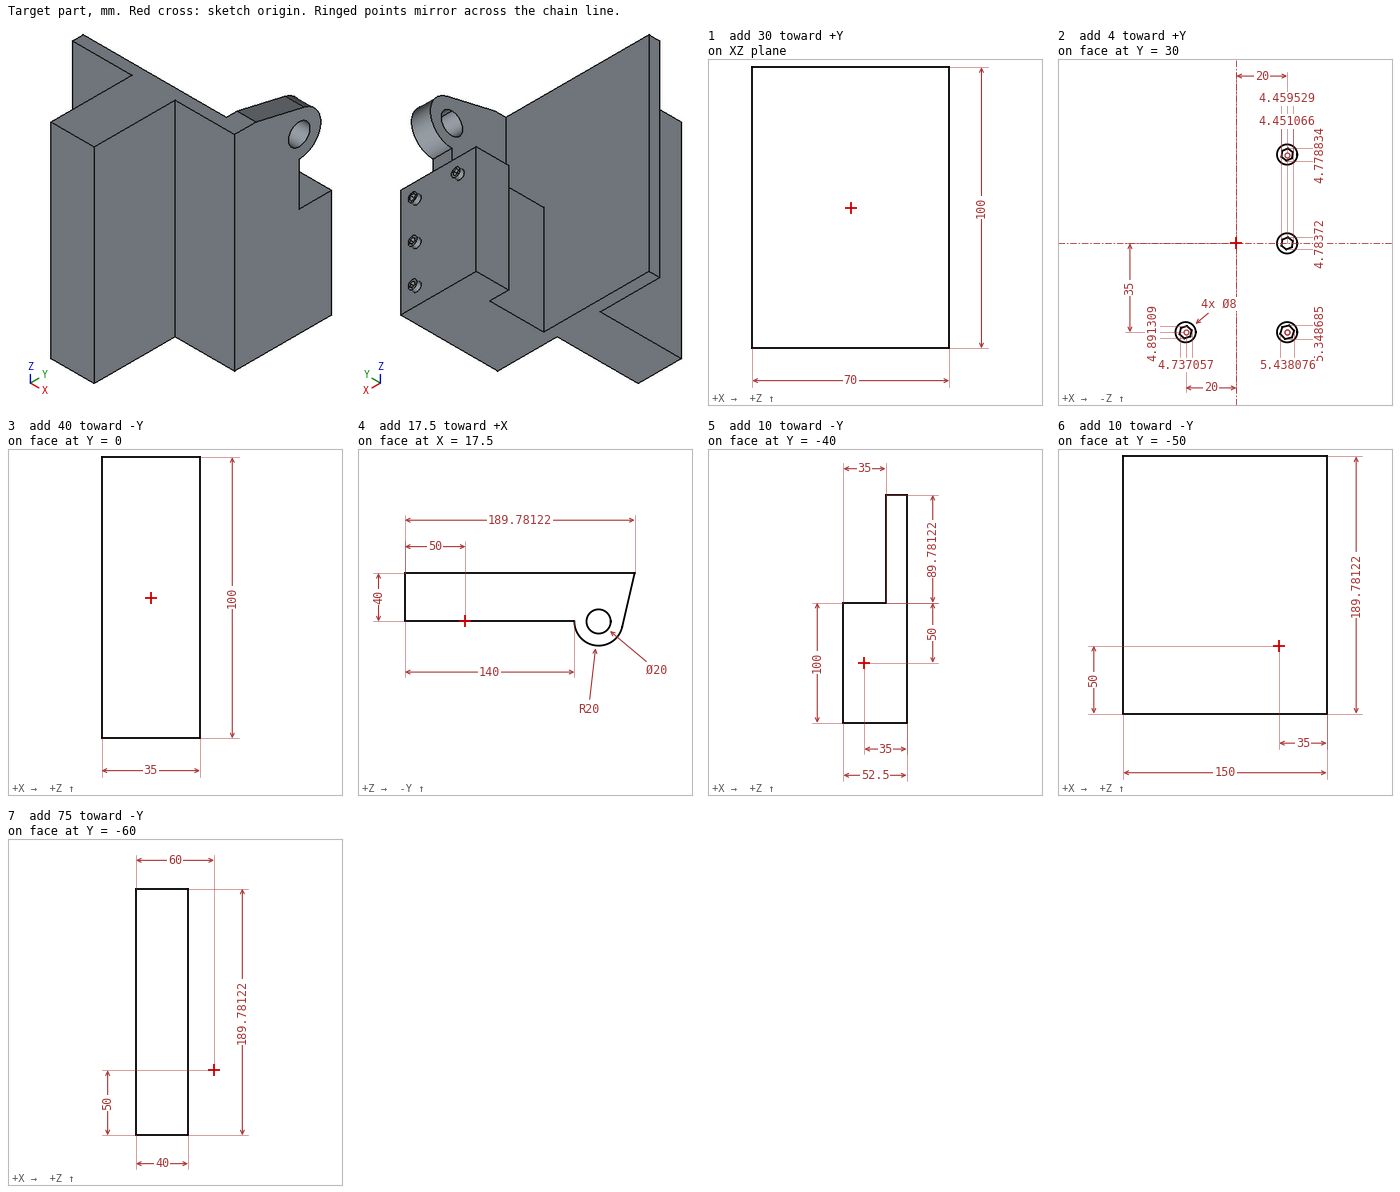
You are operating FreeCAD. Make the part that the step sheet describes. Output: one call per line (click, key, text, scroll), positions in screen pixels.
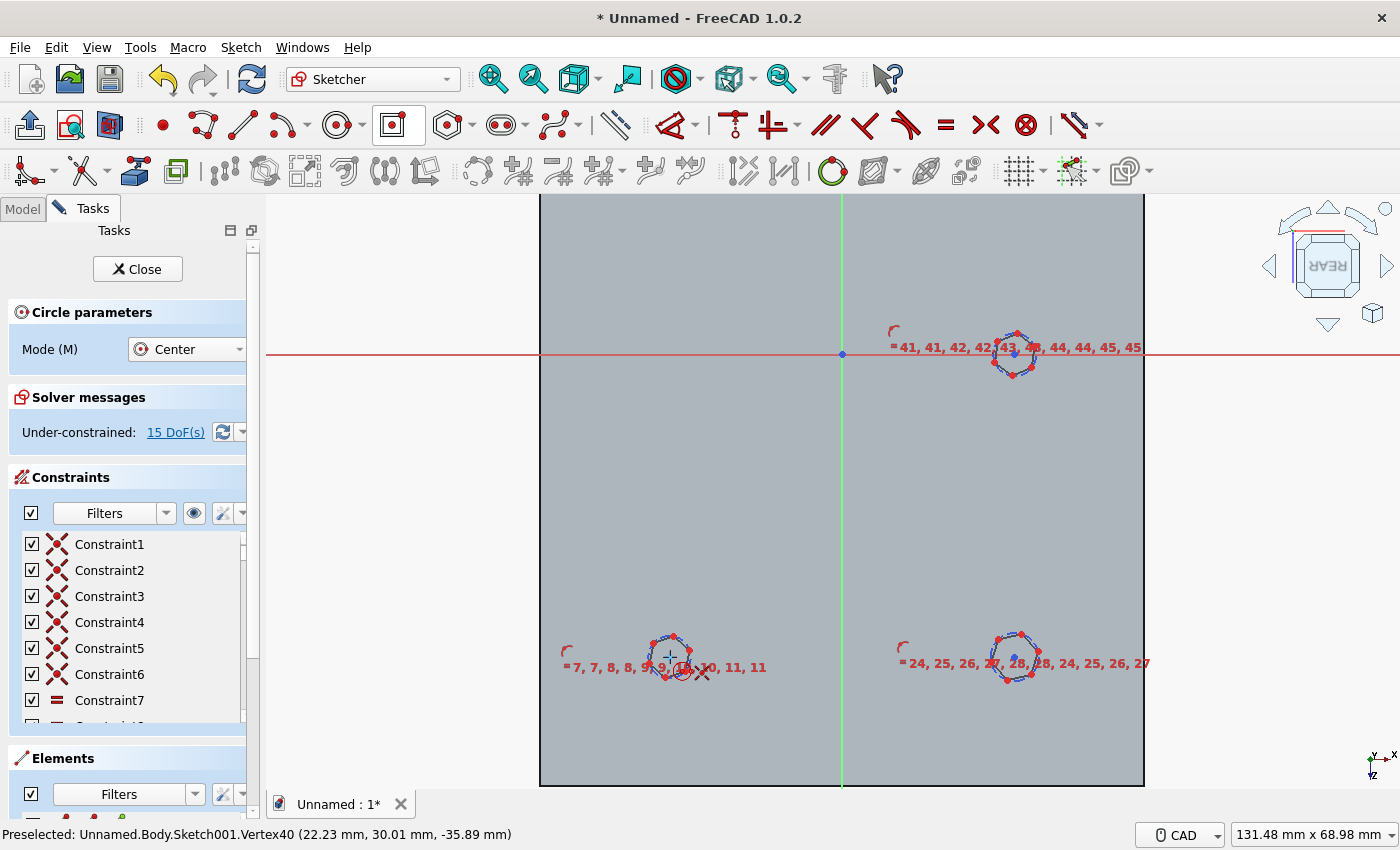
click(670, 657)
move(694, 632)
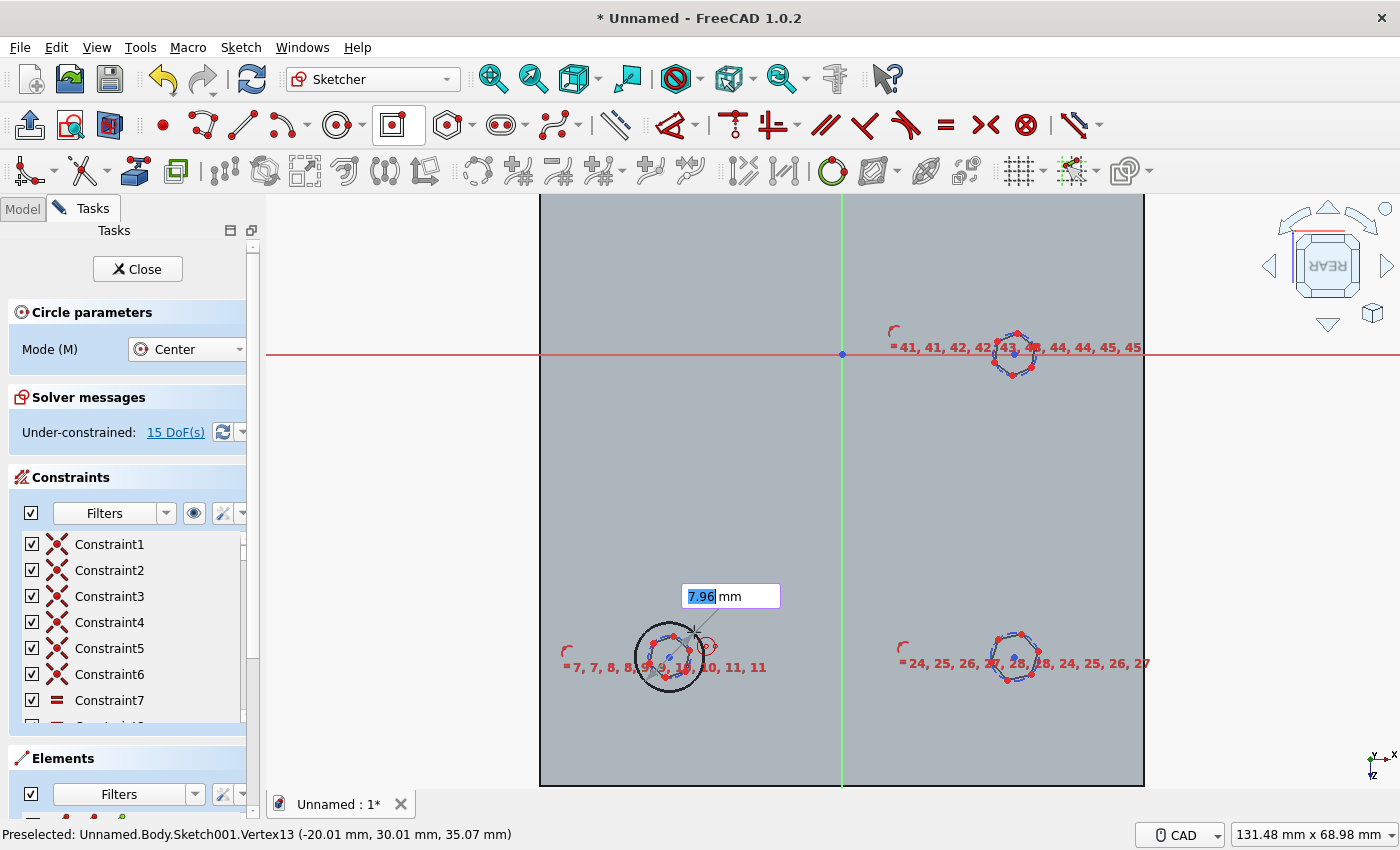
text(8)
key(Return)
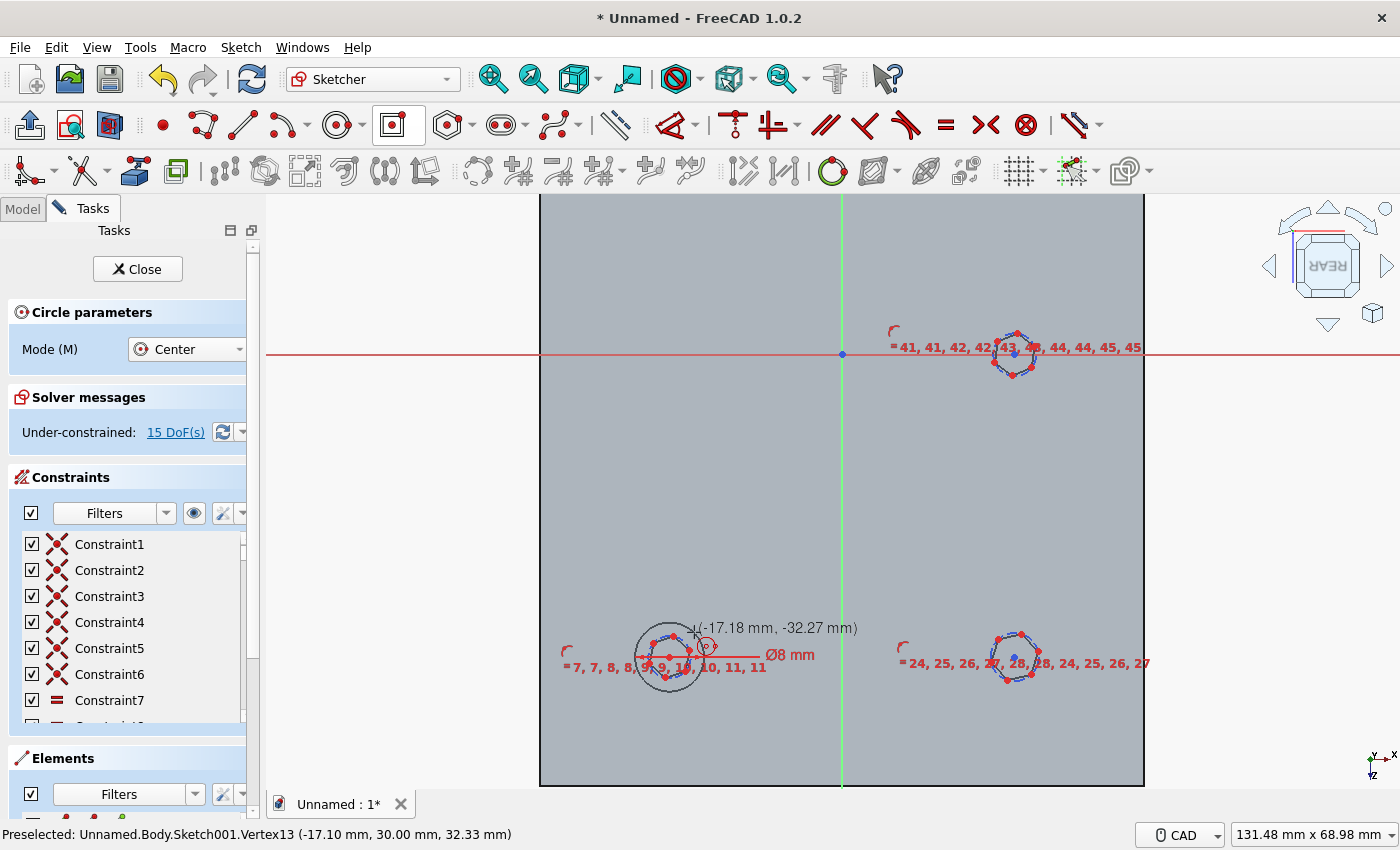
click(1015, 657)
move(1039, 632)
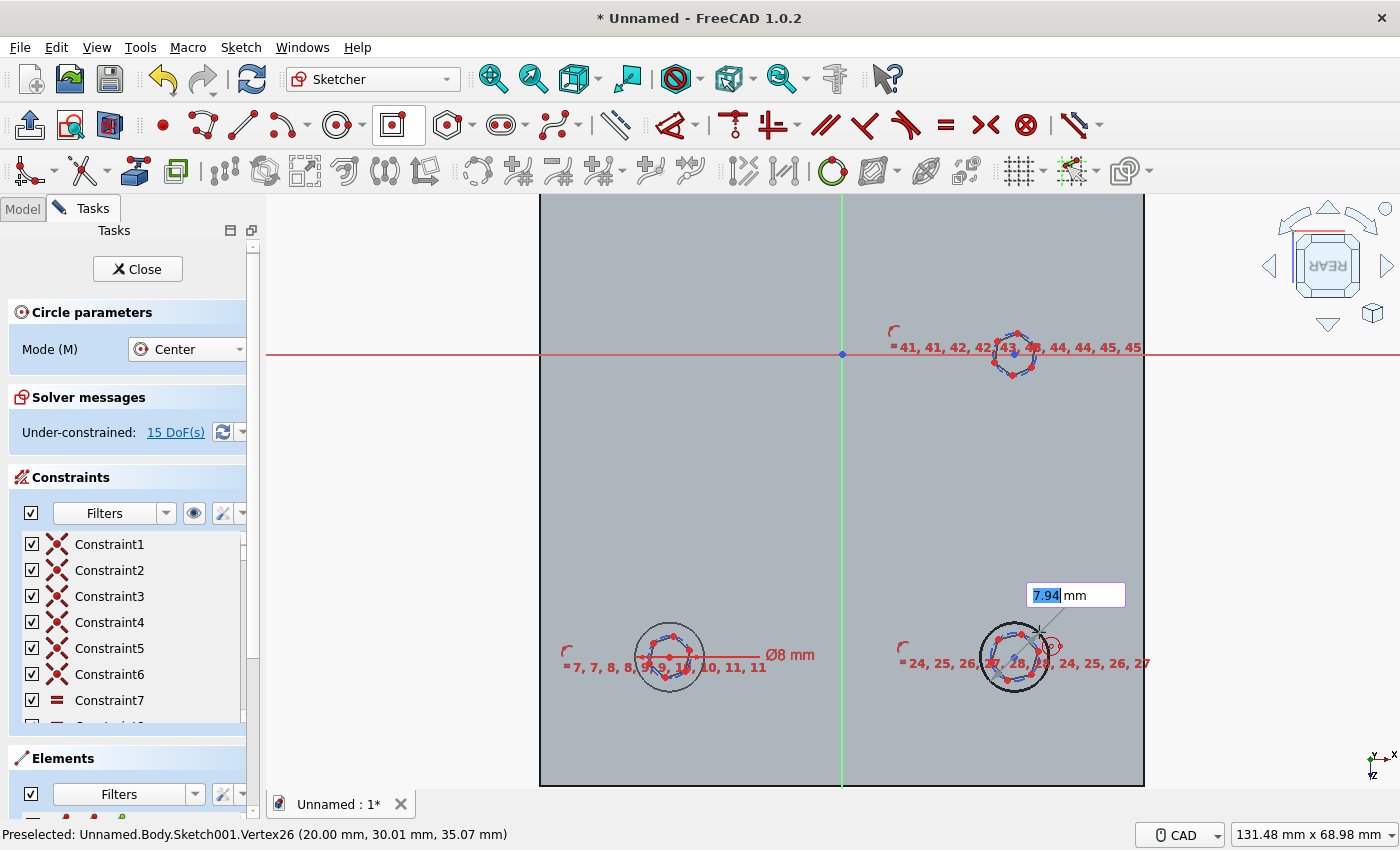
text(8)
key(Return)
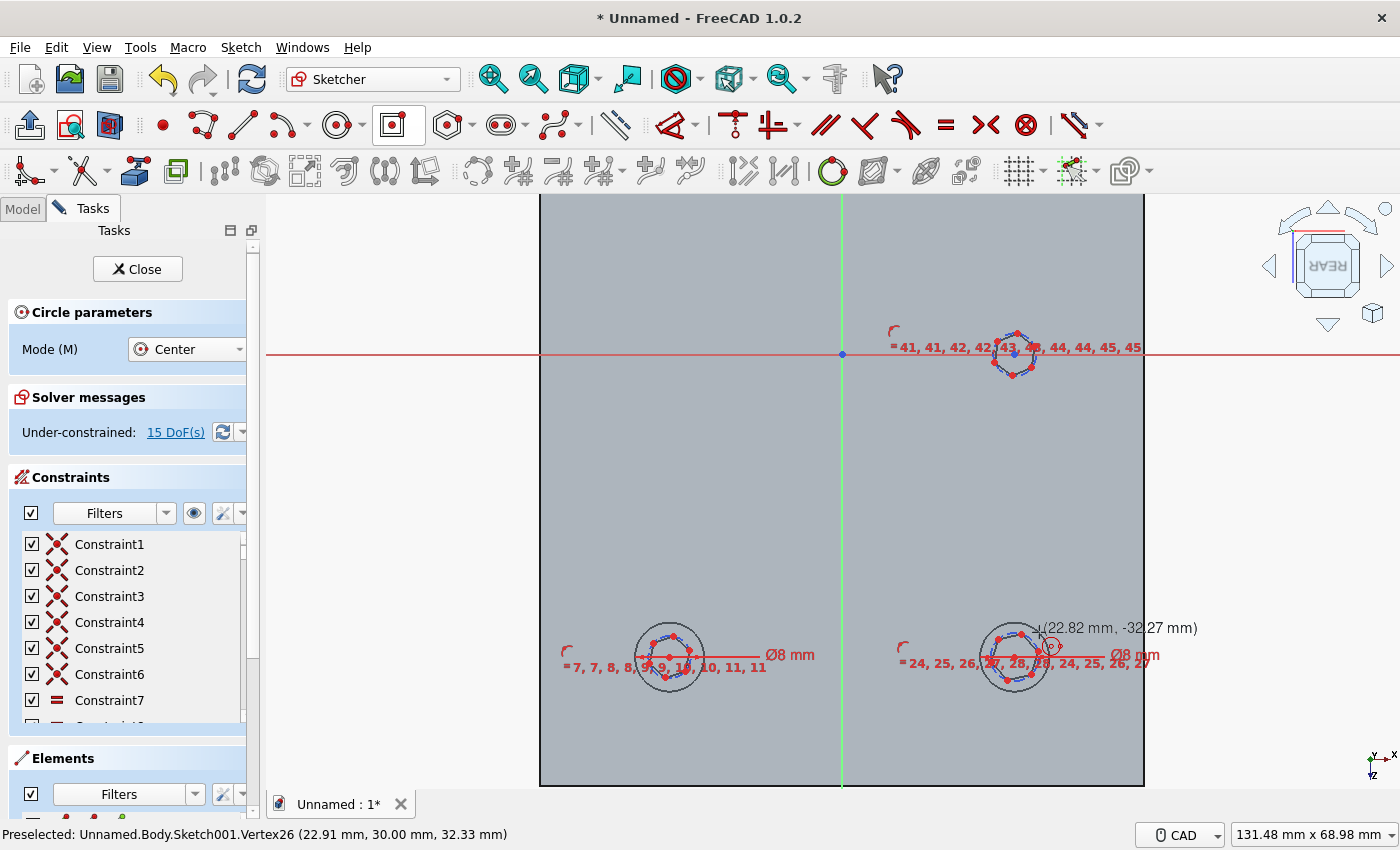
click(1015, 355)
move(1039, 330)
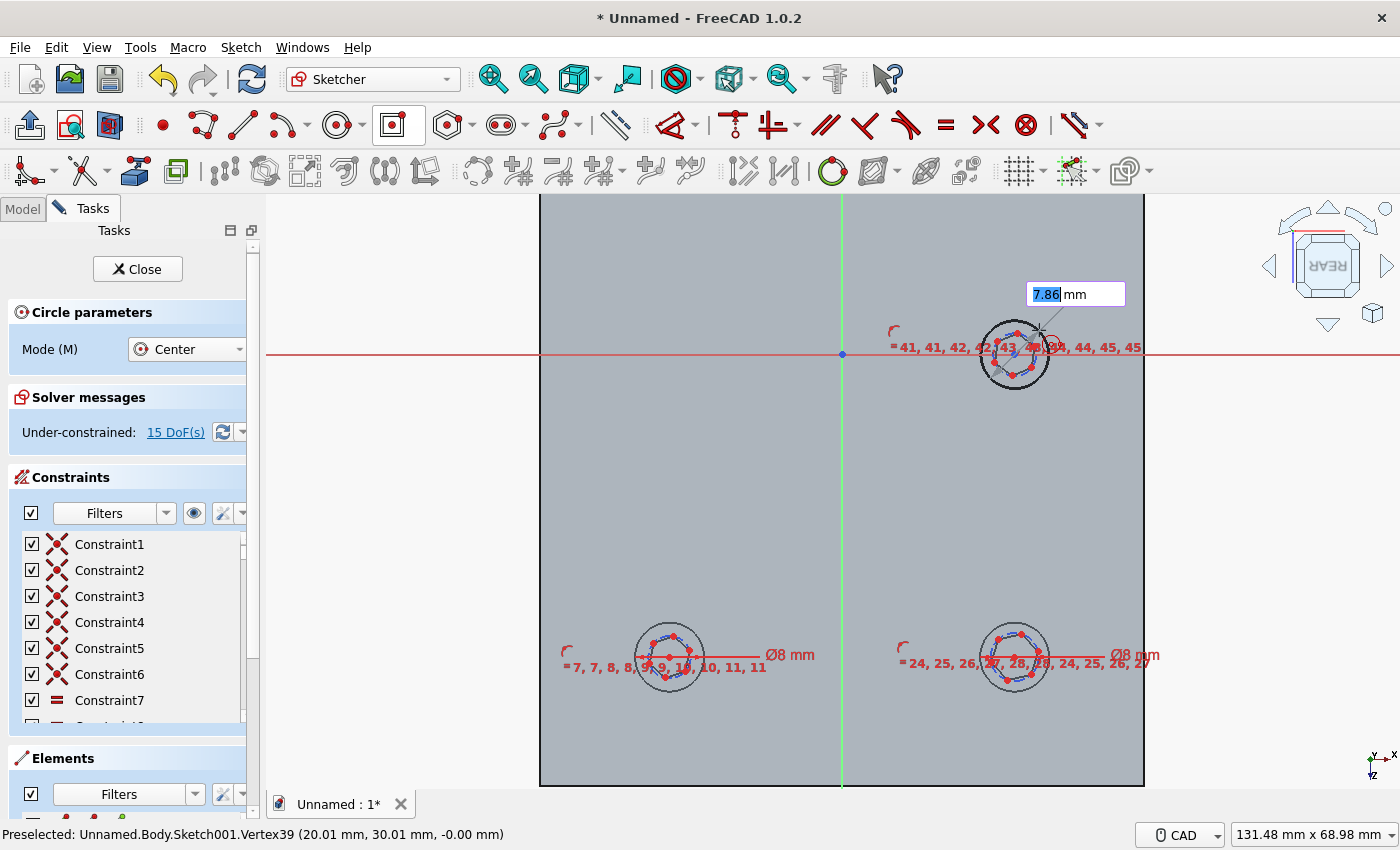
text(8)
key(Return)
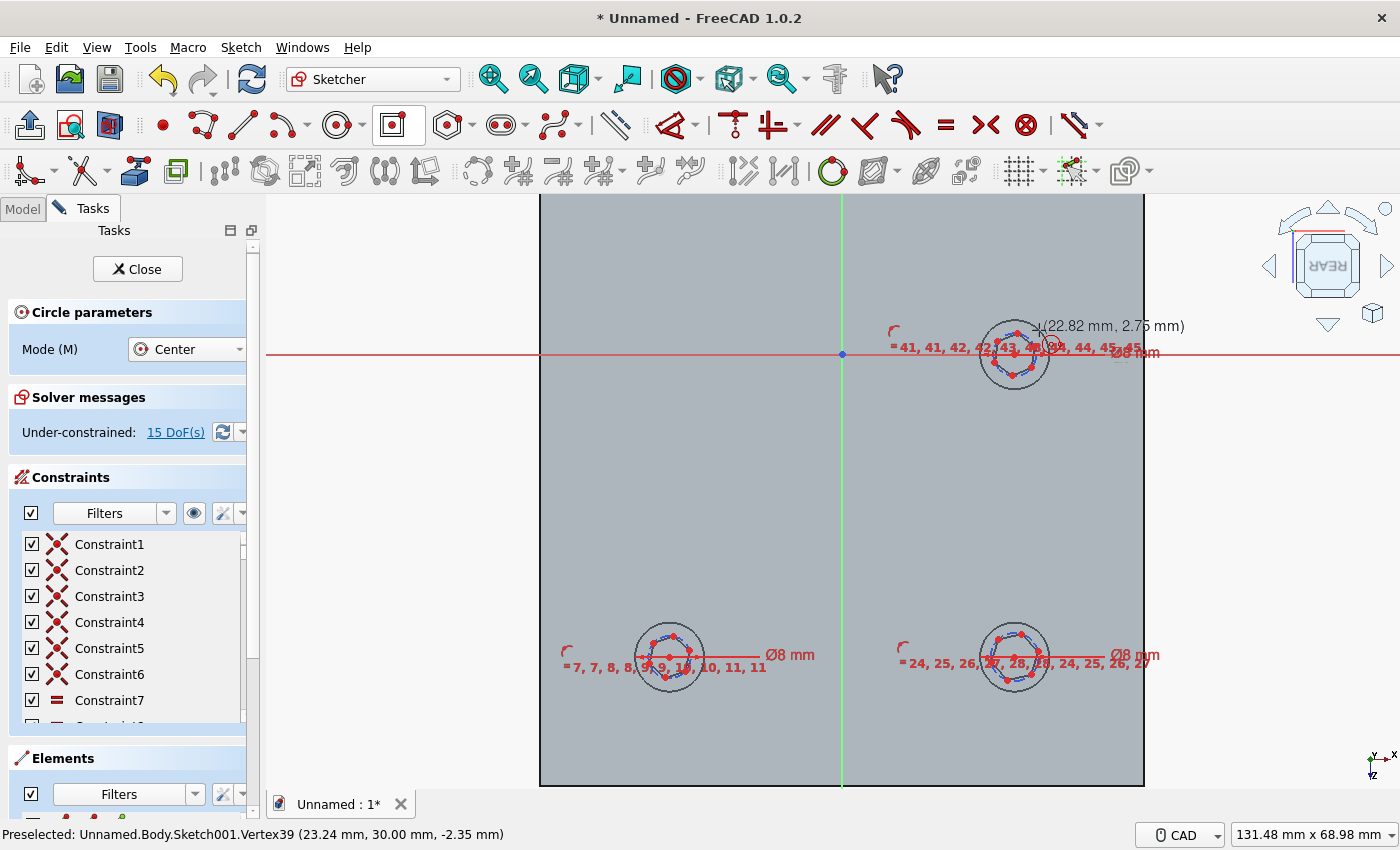
scroll(670, 658, down, 3)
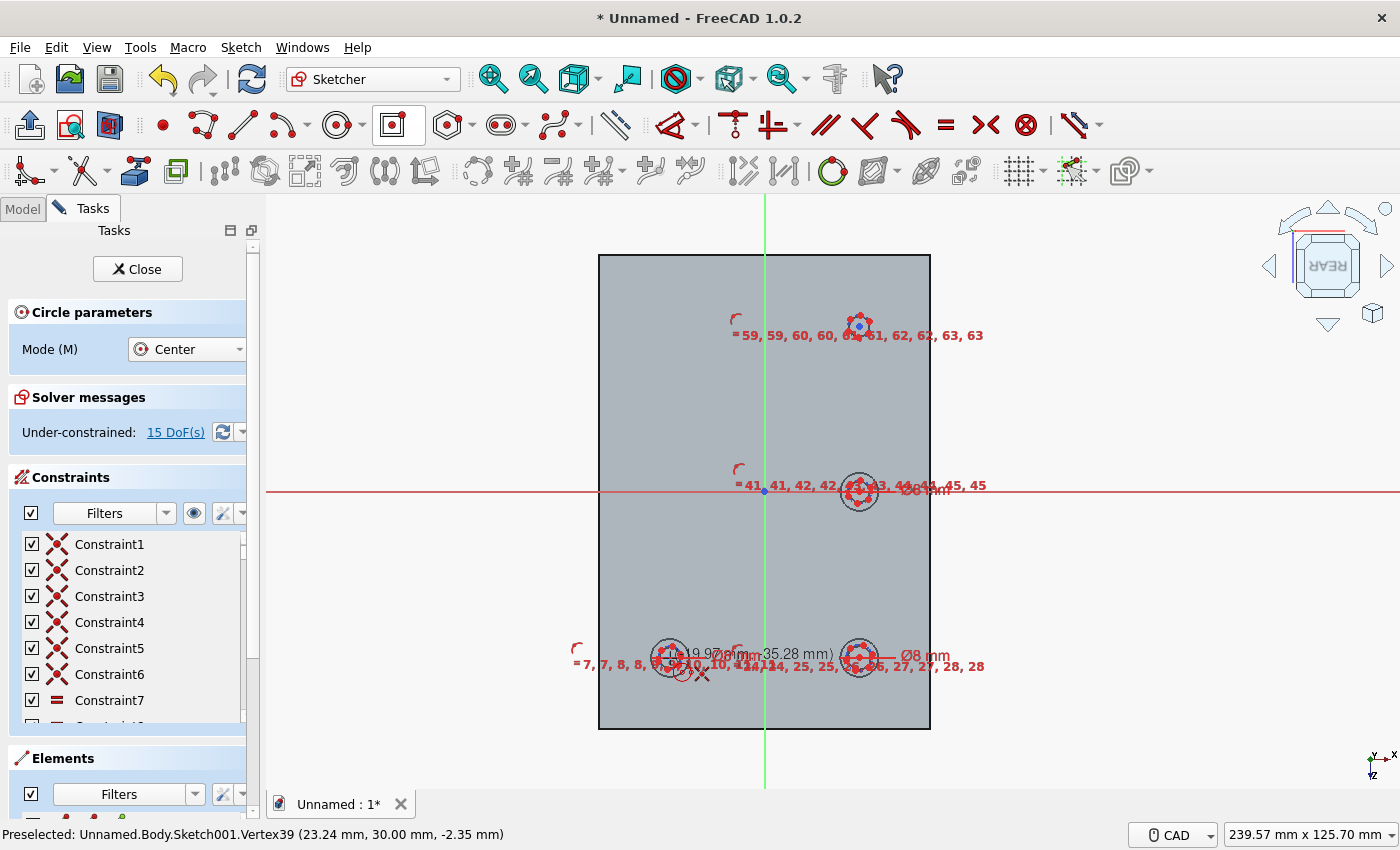
scroll(859, 326, up, 3)